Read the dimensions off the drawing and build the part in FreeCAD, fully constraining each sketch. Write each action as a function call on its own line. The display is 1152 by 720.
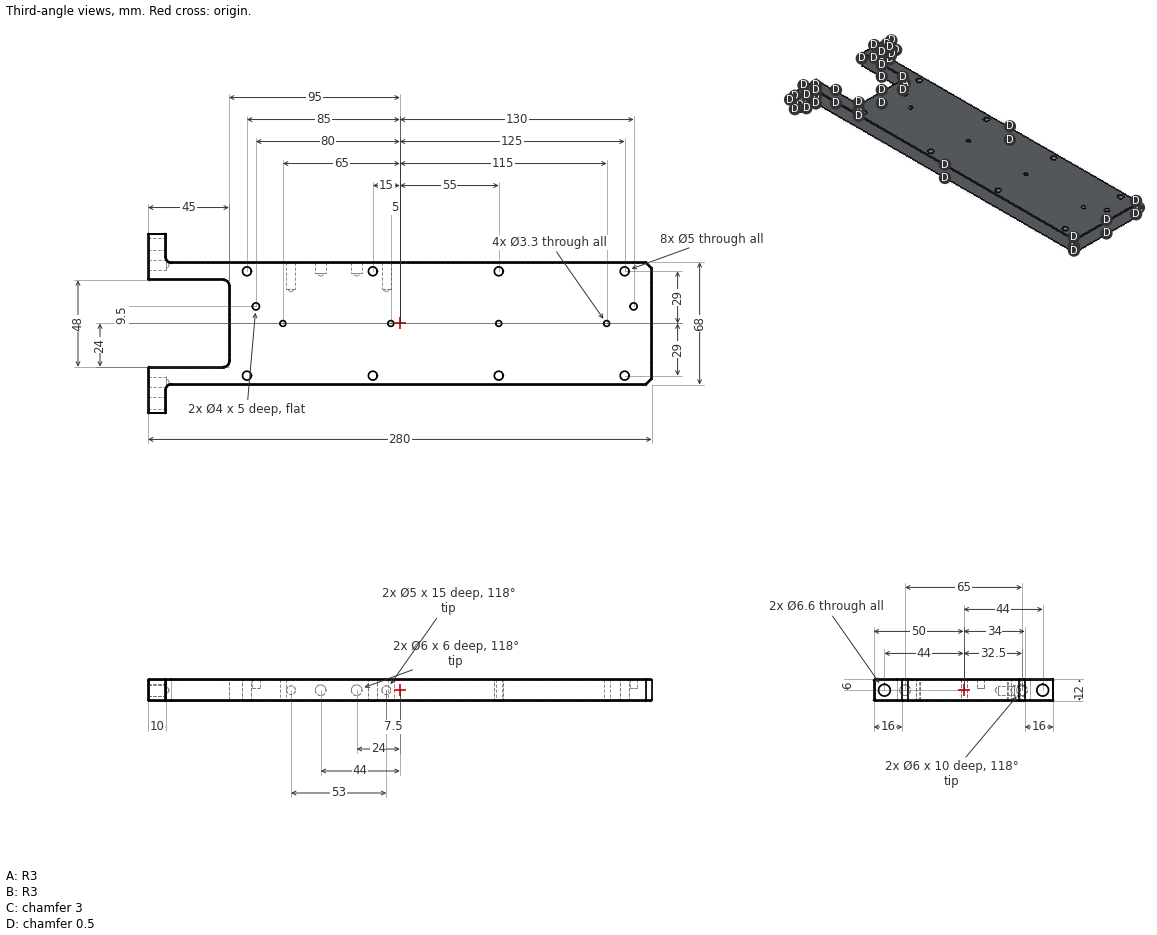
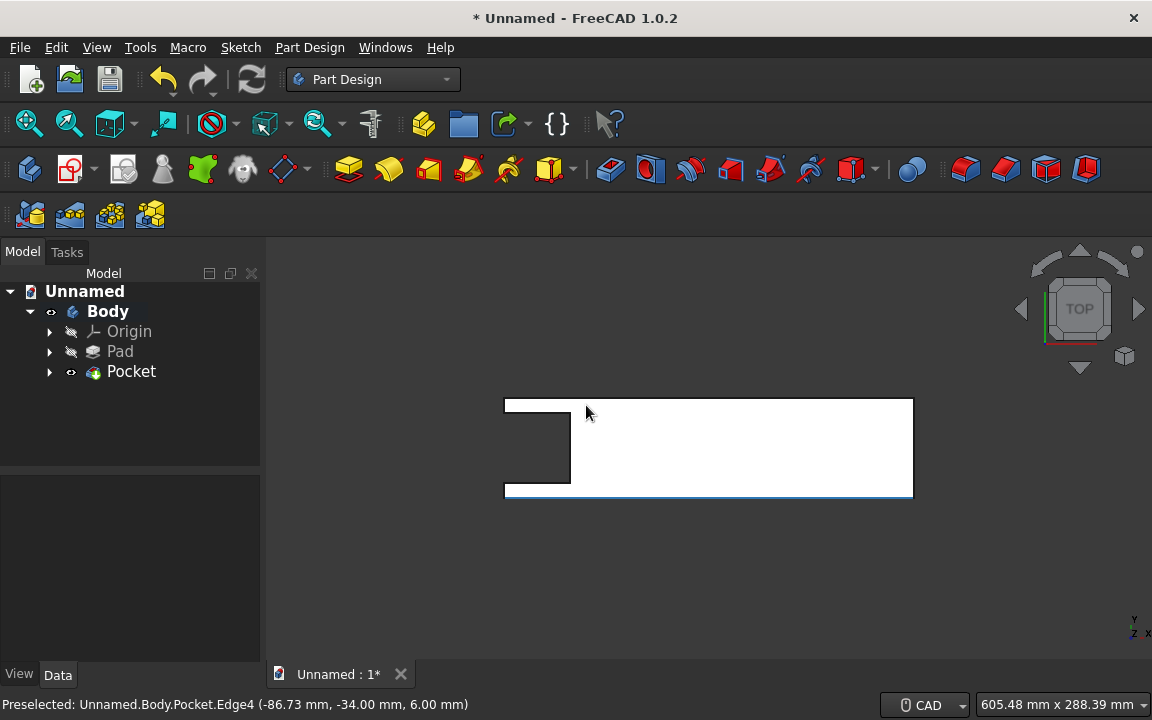
scroll(570, 482, up, 5)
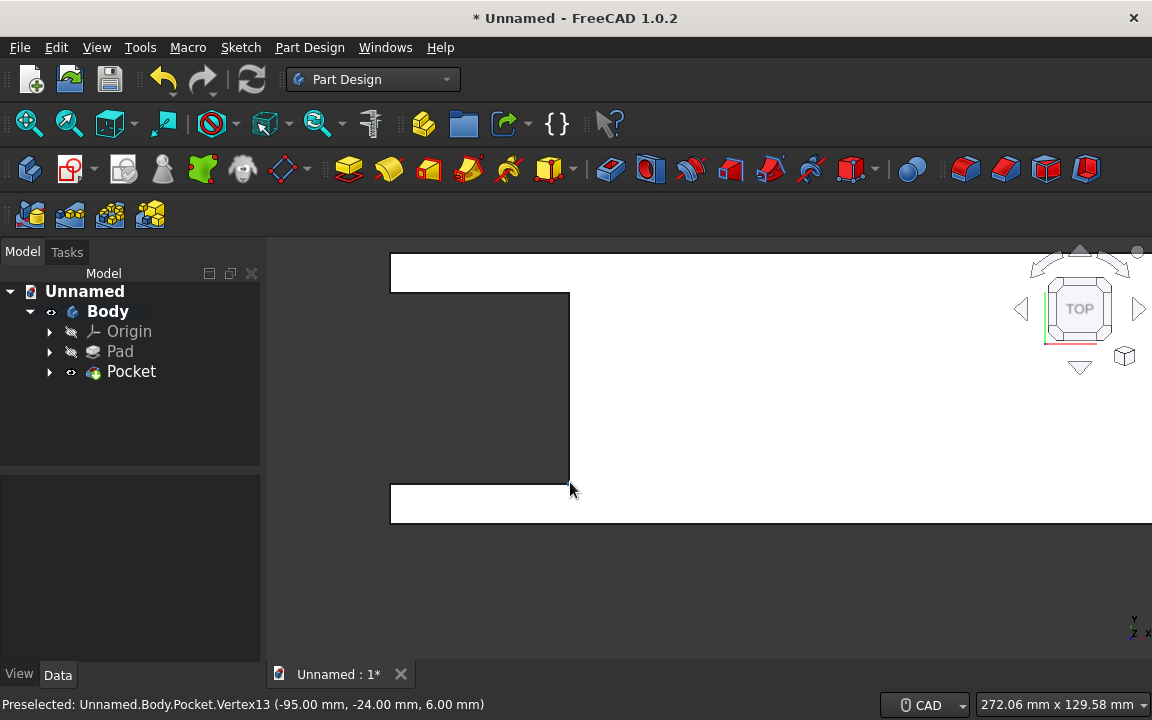
key(v)
key(f)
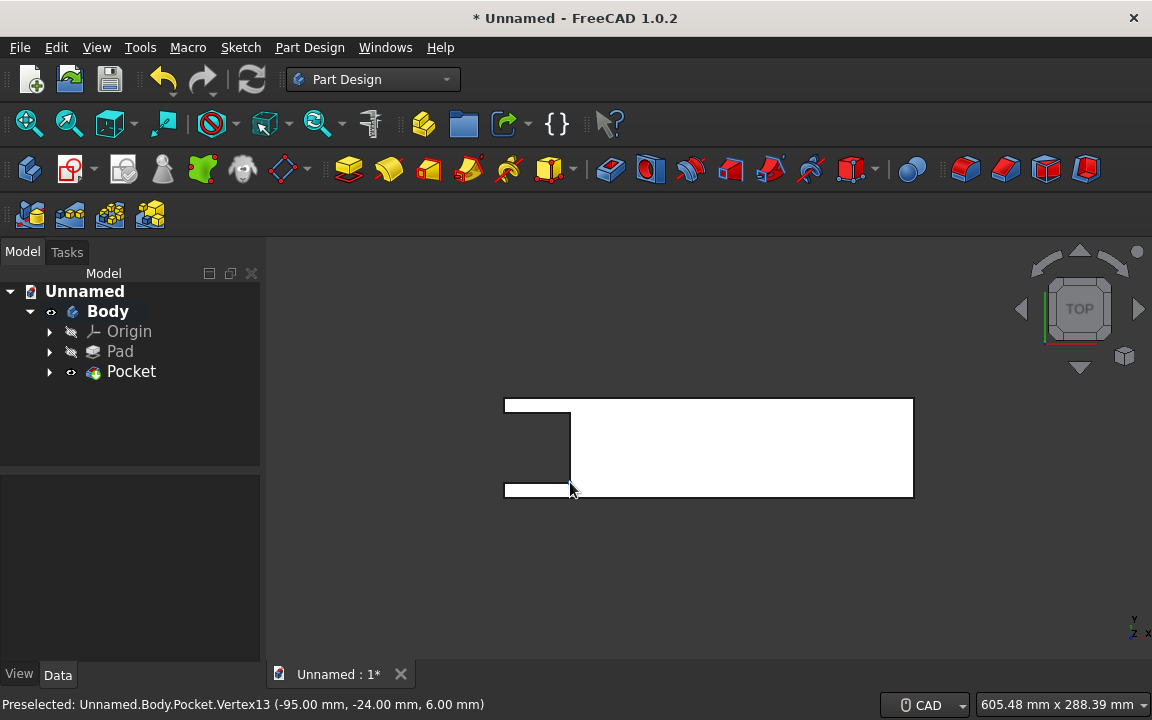
key(1)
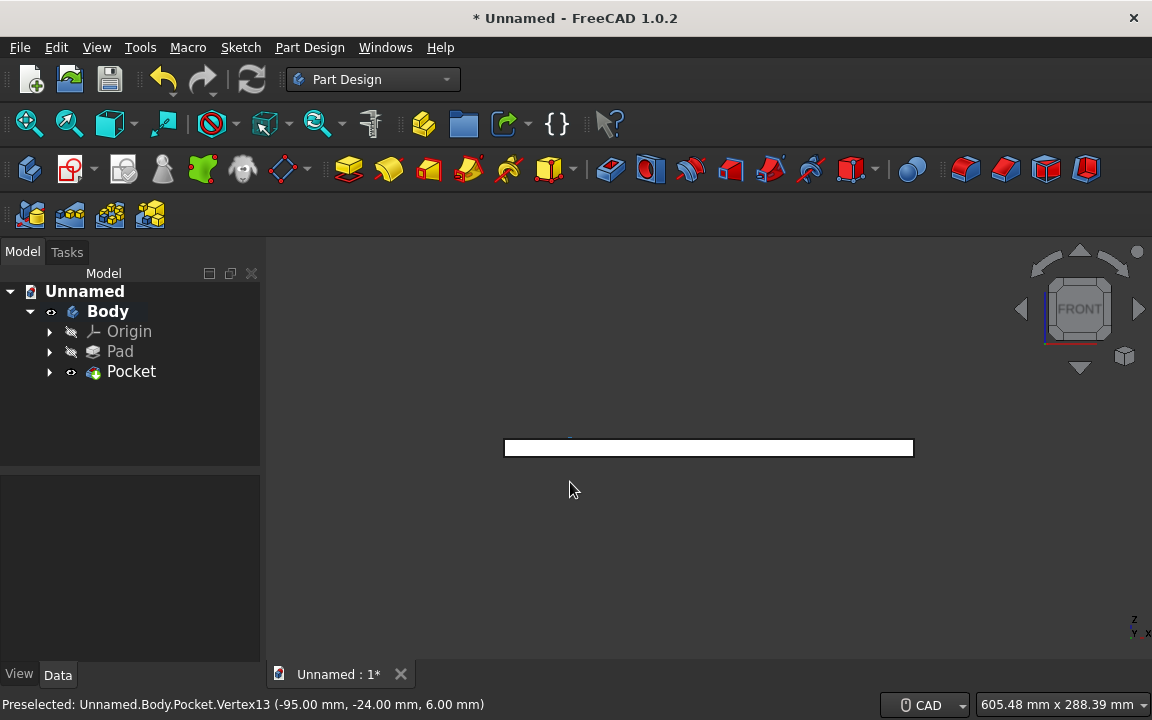
scroll(570, 447, up, 5)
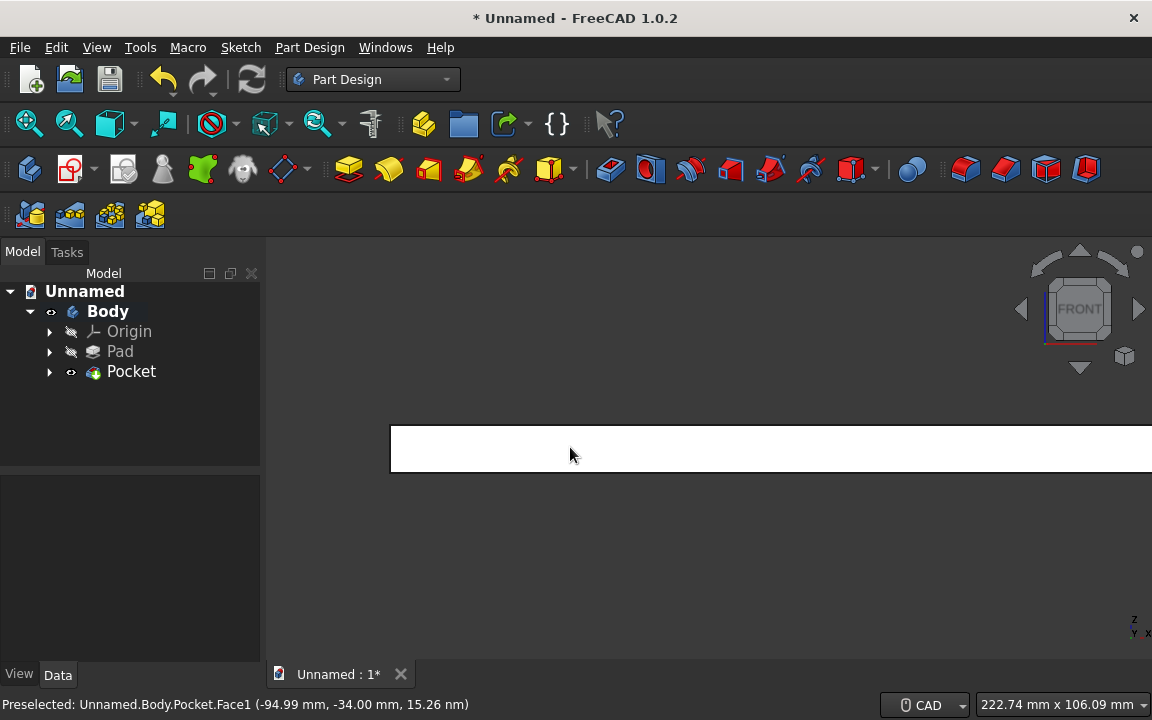
click(30, 124)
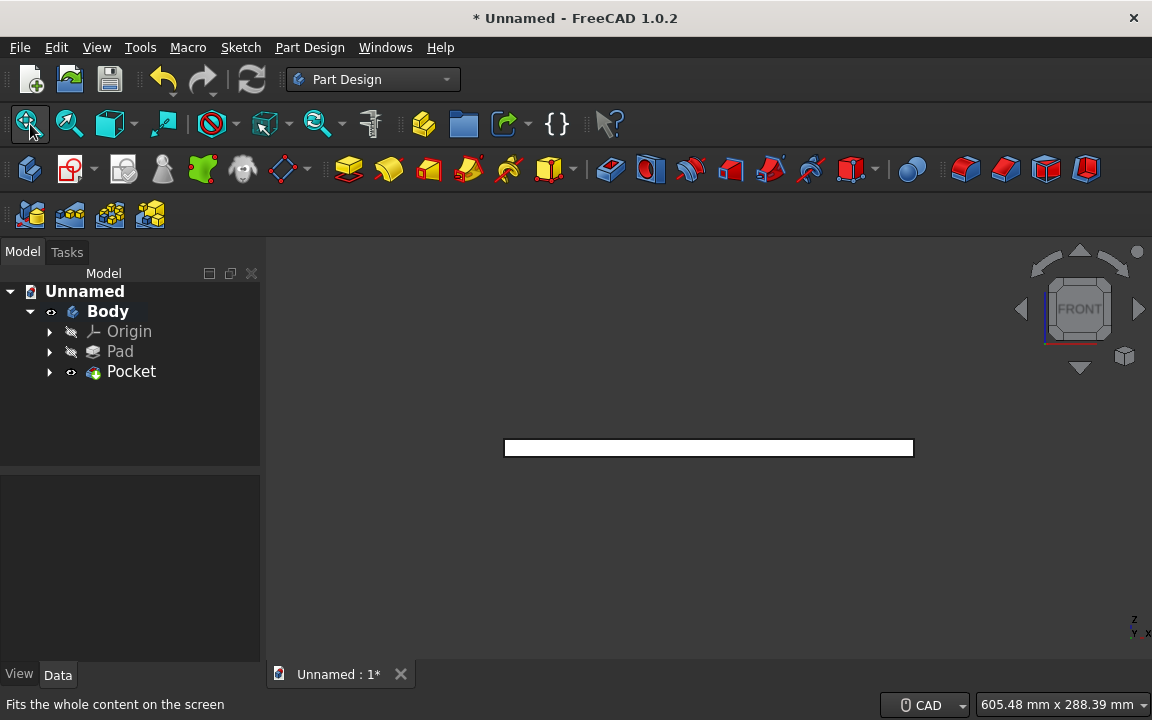
key(3)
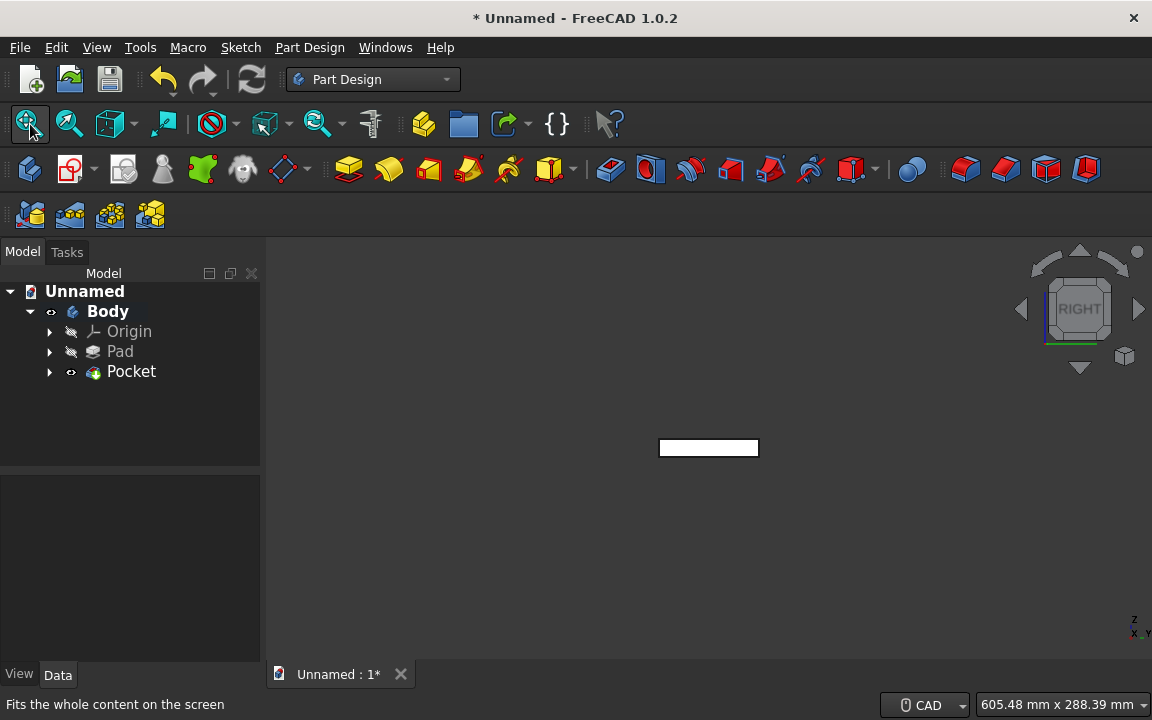
click(30, 124)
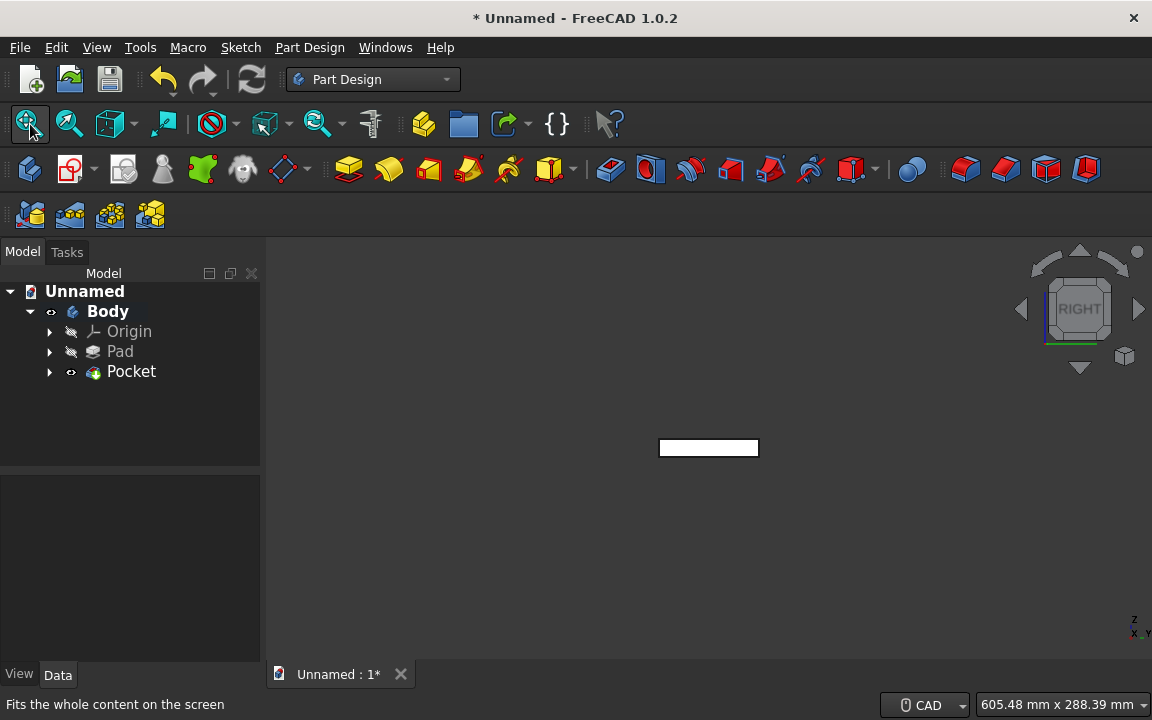
scroll(674, 447, up, 5)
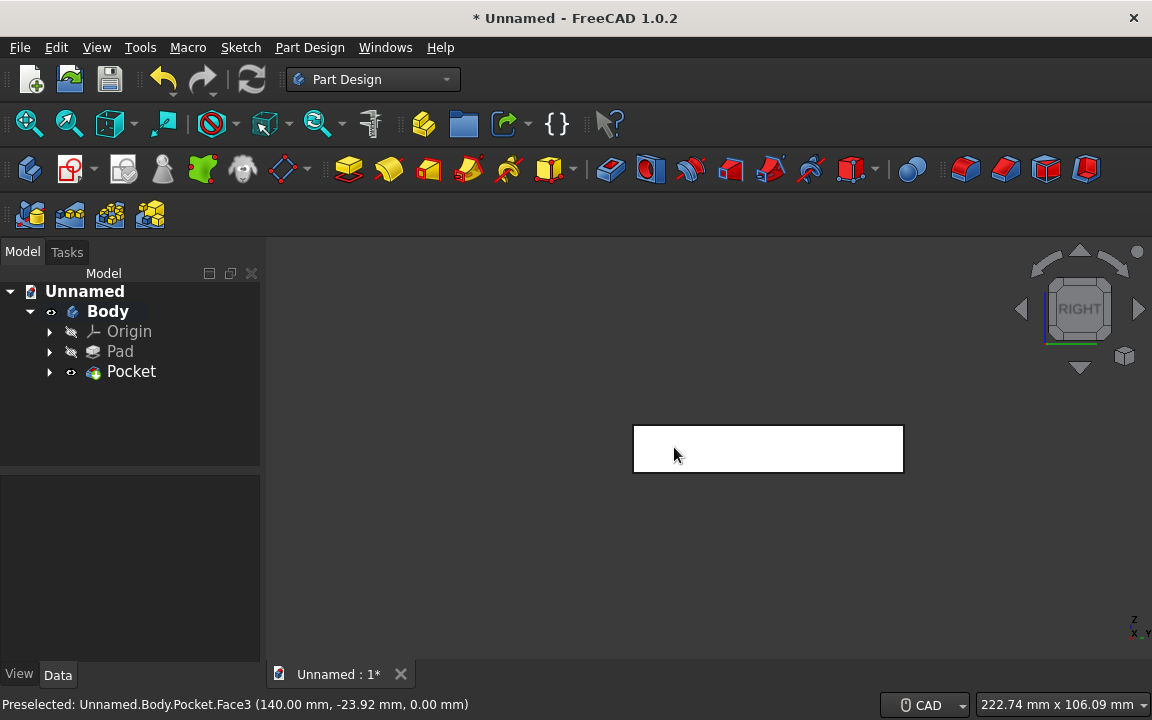
key(v)
key(f)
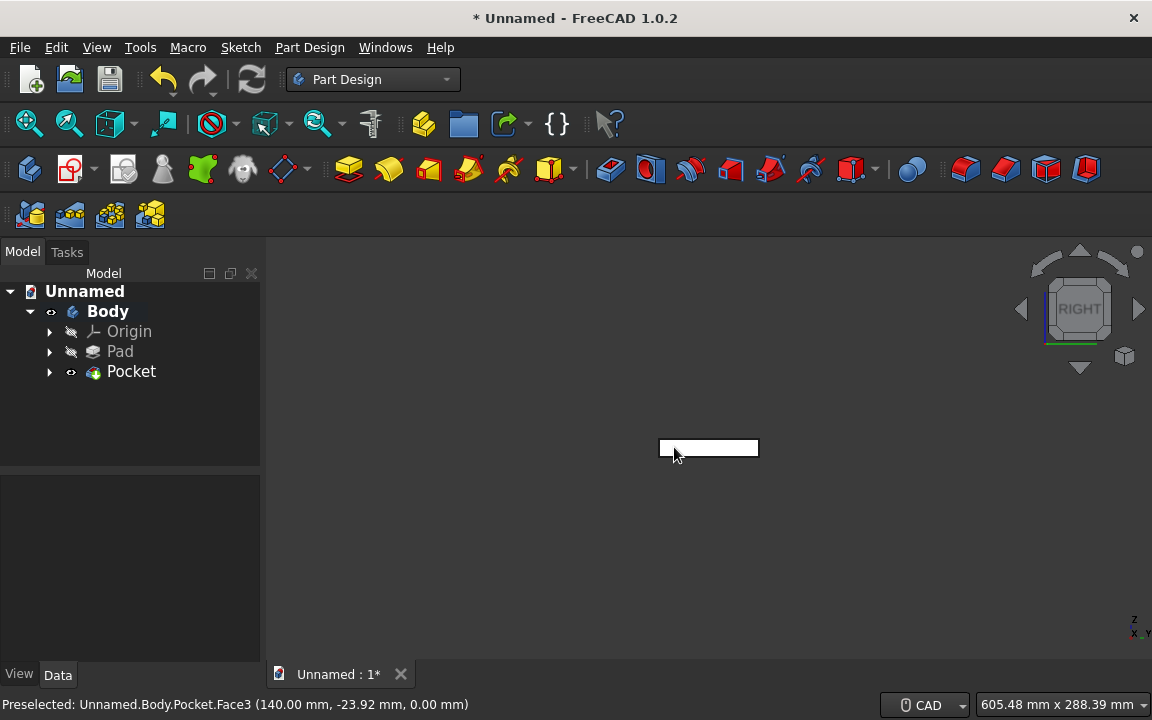
key(5)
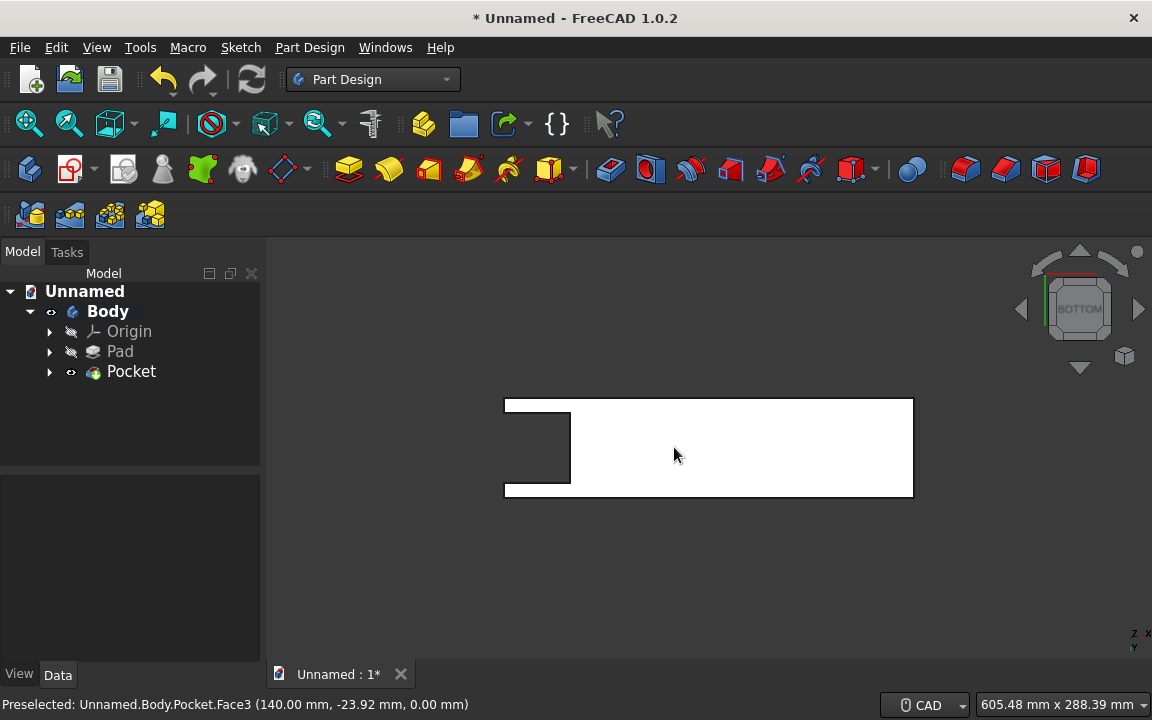
scroll(570, 412, up, 5)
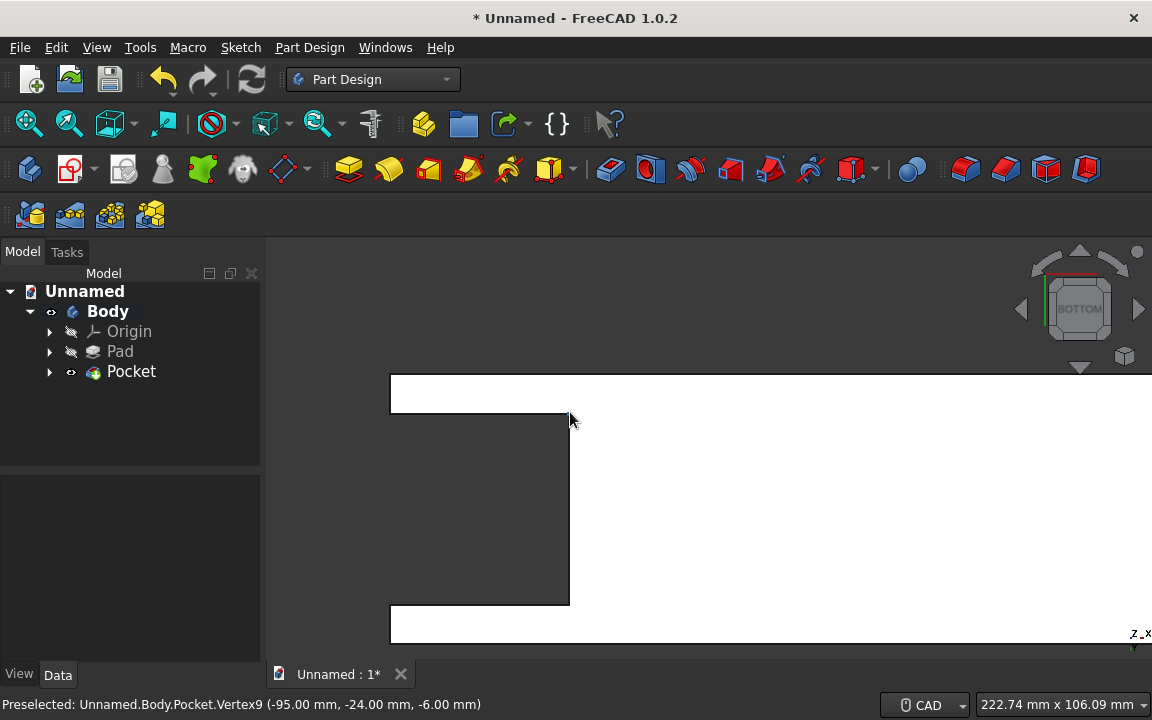
key(v)
key(f)